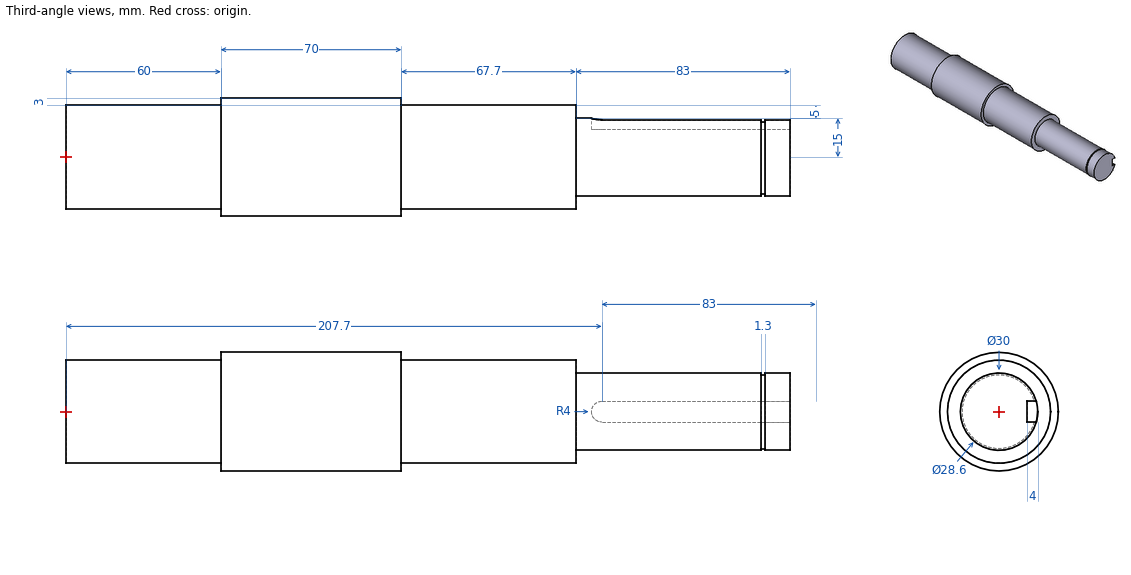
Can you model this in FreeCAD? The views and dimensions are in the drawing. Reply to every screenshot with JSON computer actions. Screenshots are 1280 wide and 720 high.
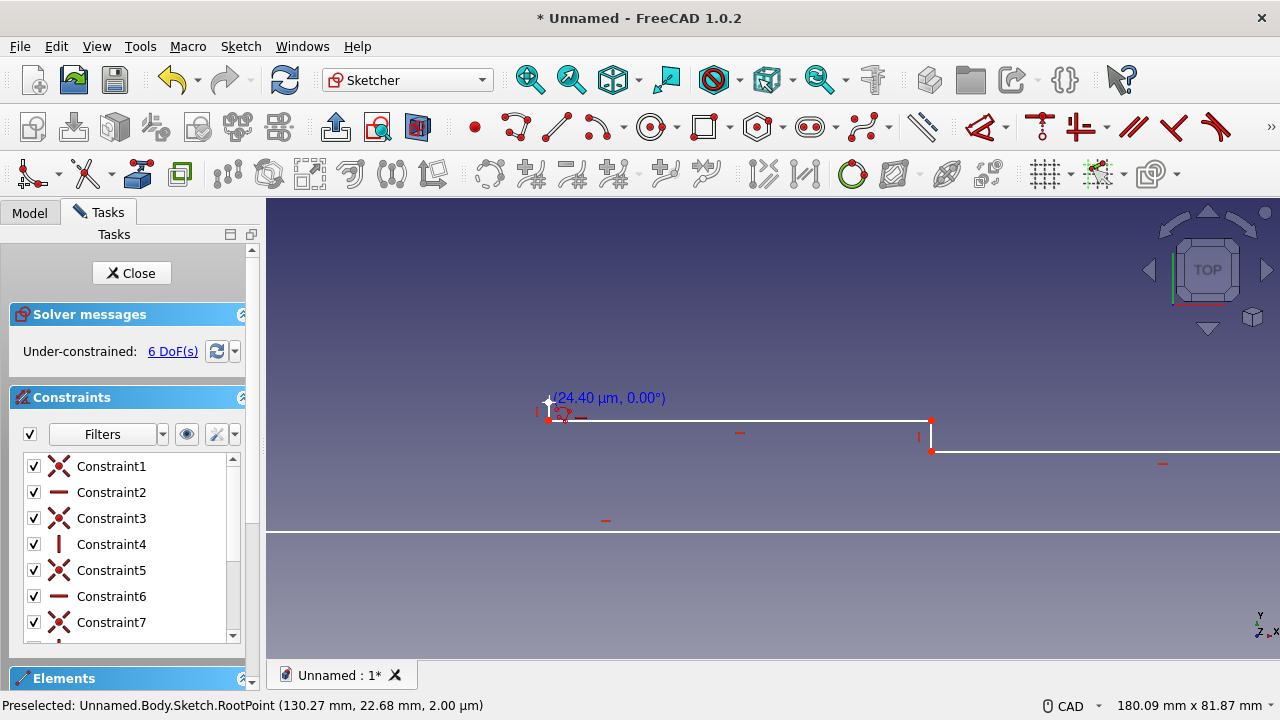
{"action": "scroll", "coordinate": [761, 406], "scroll_direction": "down", "scroll_amount": 5}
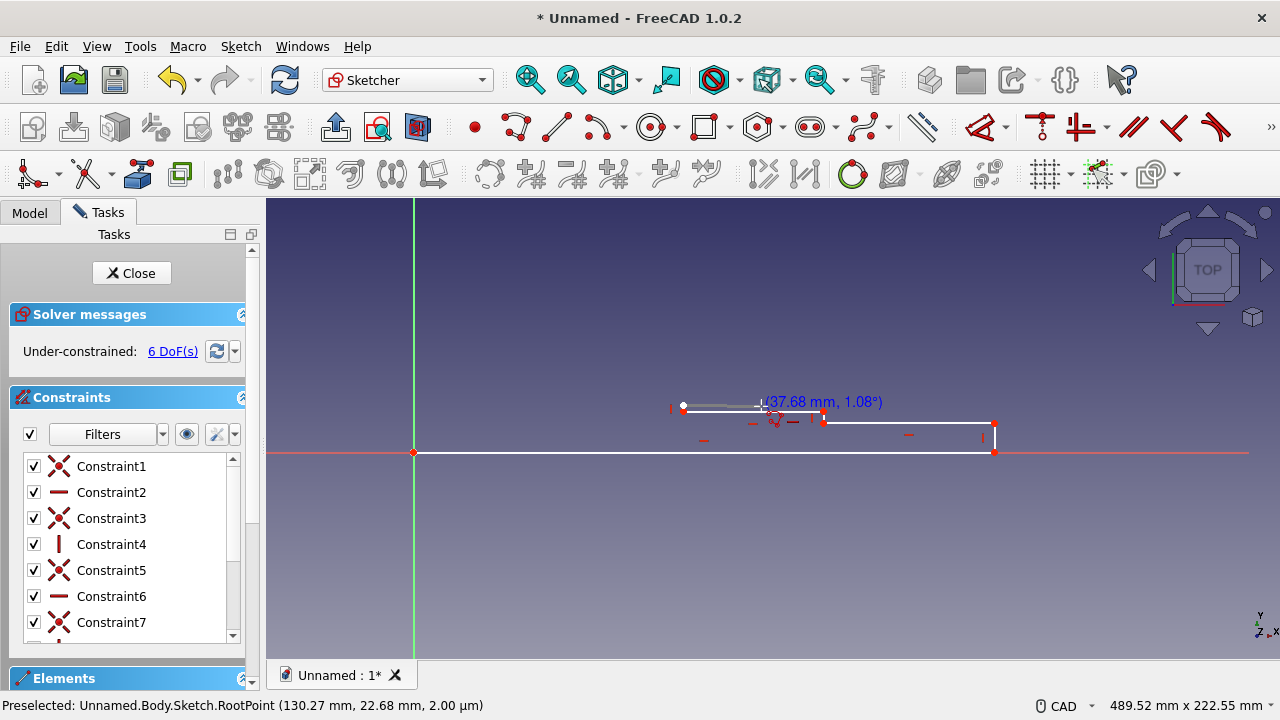
{"action": "left_click", "coordinate": [538, 405]}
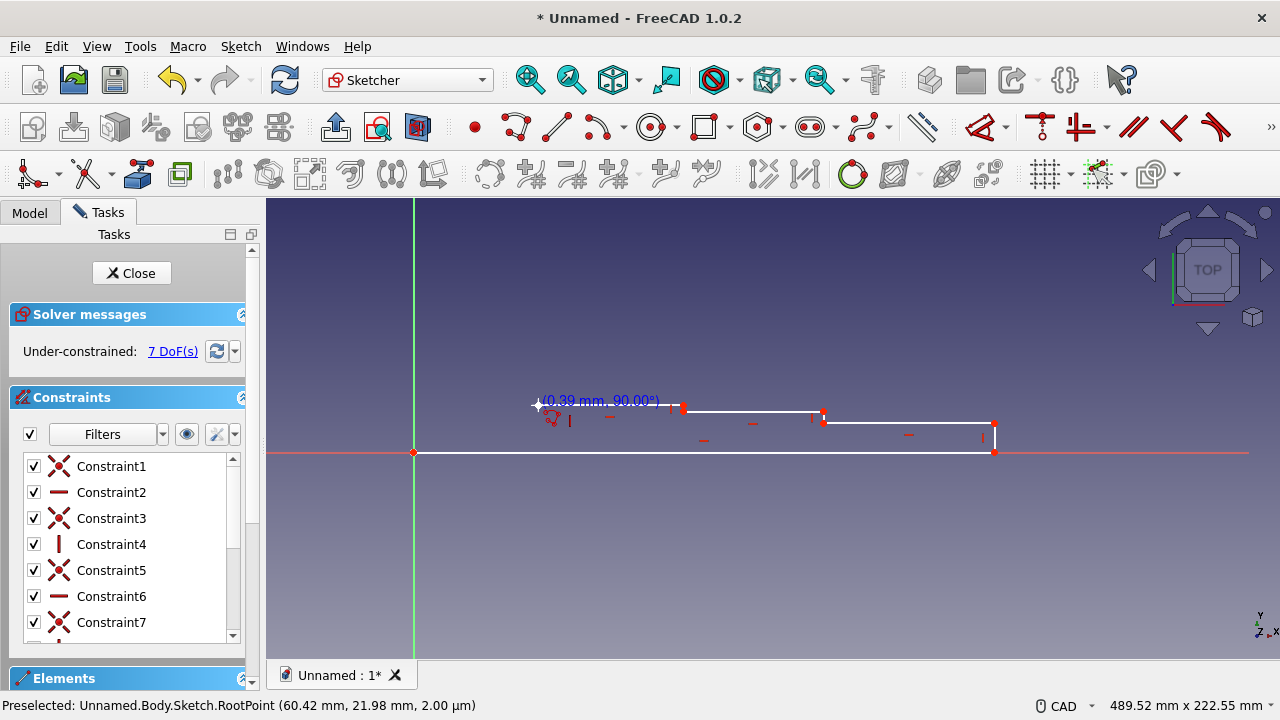
{"action": "scroll", "coordinate": [538, 411], "scroll_direction": "up", "scroll_amount": 5}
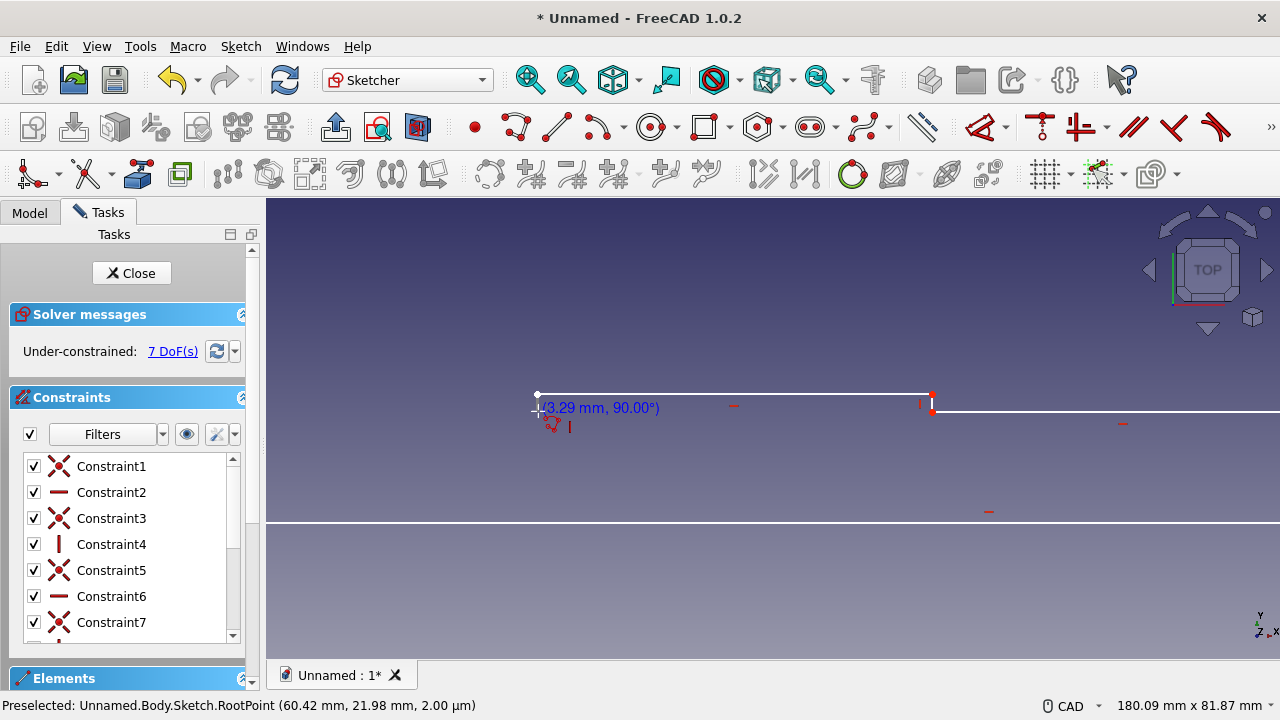
{"action": "left_click", "coordinate": [538, 410]}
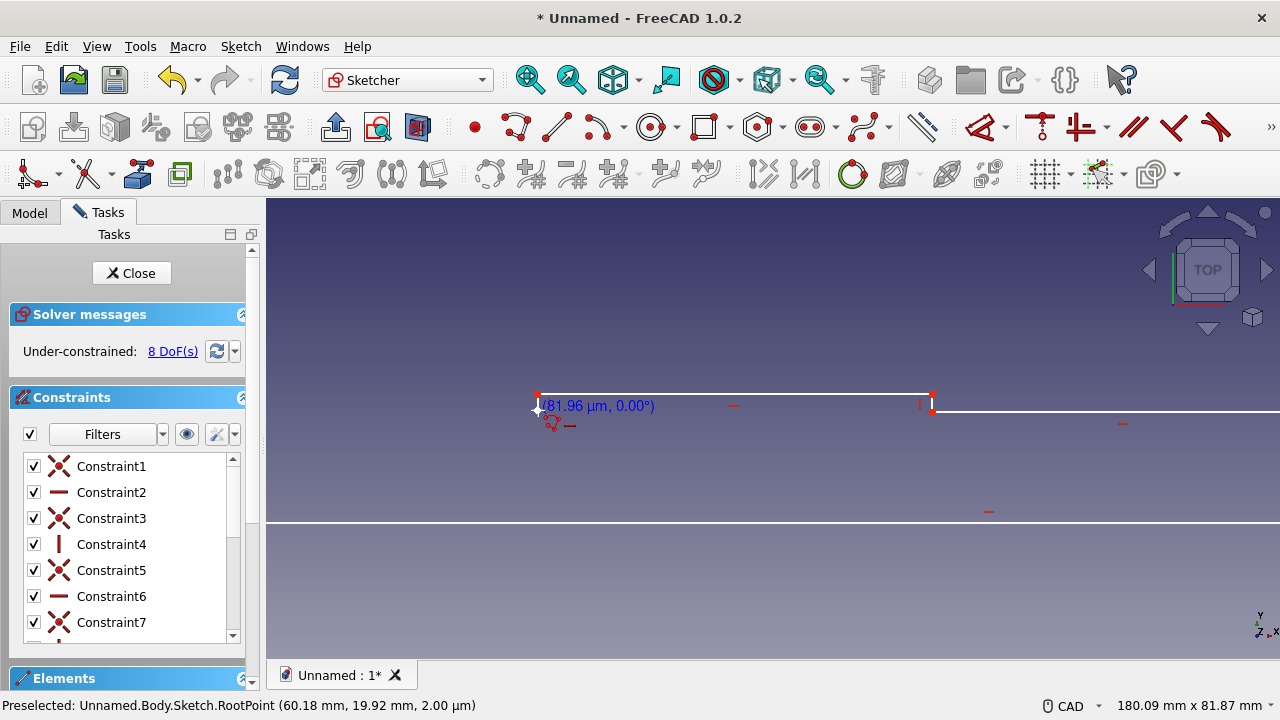
{"action": "scroll", "coordinate": [538, 411], "scroll_direction": "down", "scroll_amount": 5}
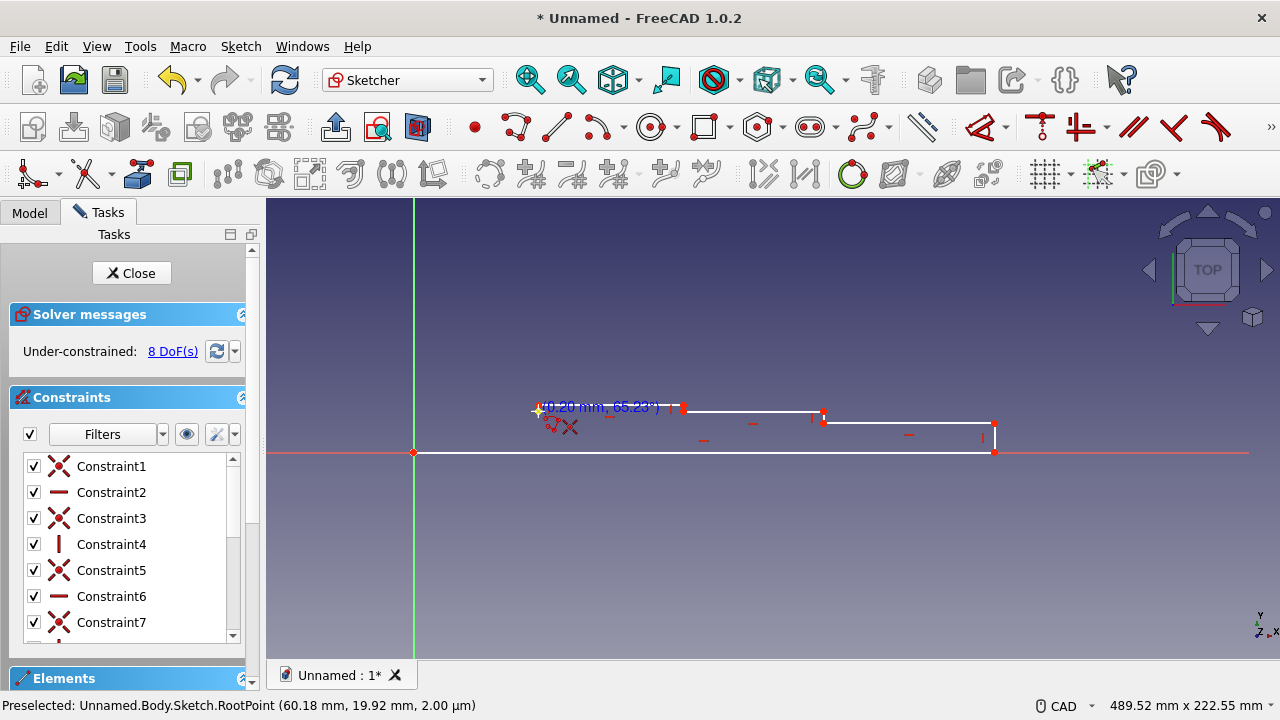
{"action": "left_click", "coordinate": [423, 411]}
{"action": "left_click", "coordinate": [414, 453]}
{"action": "key", "text": "Escape"}
{"action": "key", "text": "Escape"}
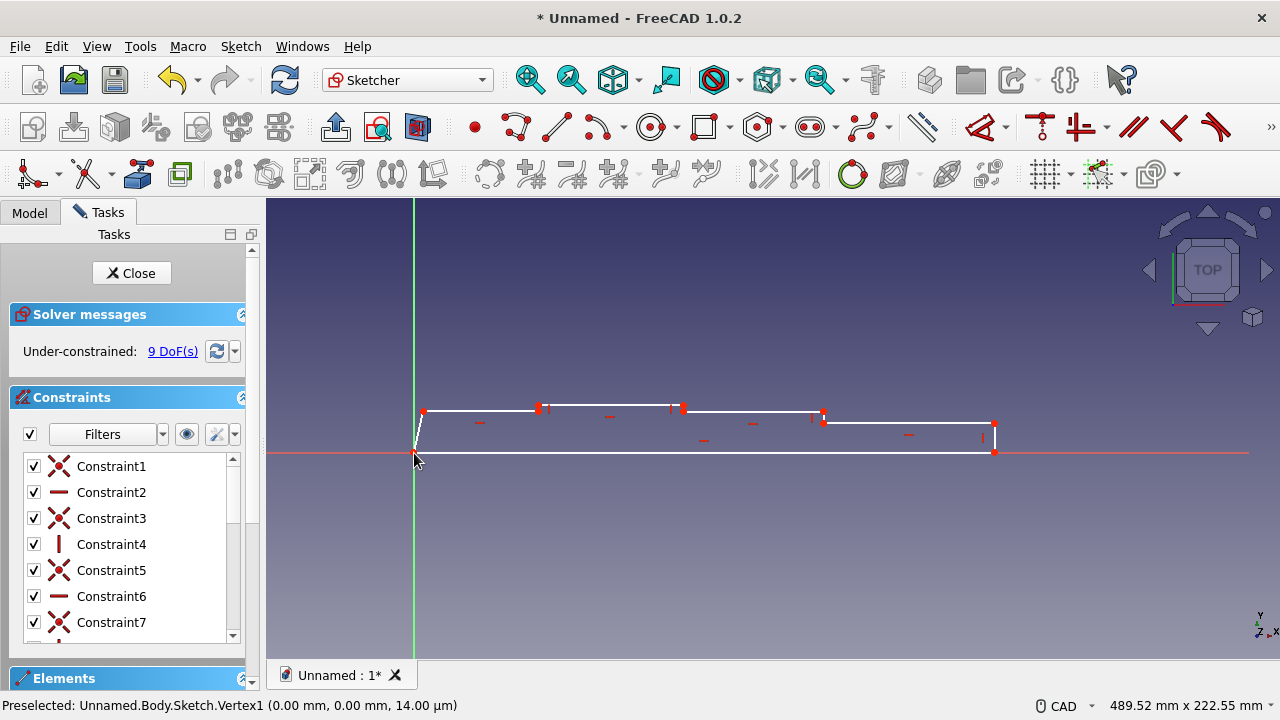
{"action": "left_click", "coordinate": [417, 440]}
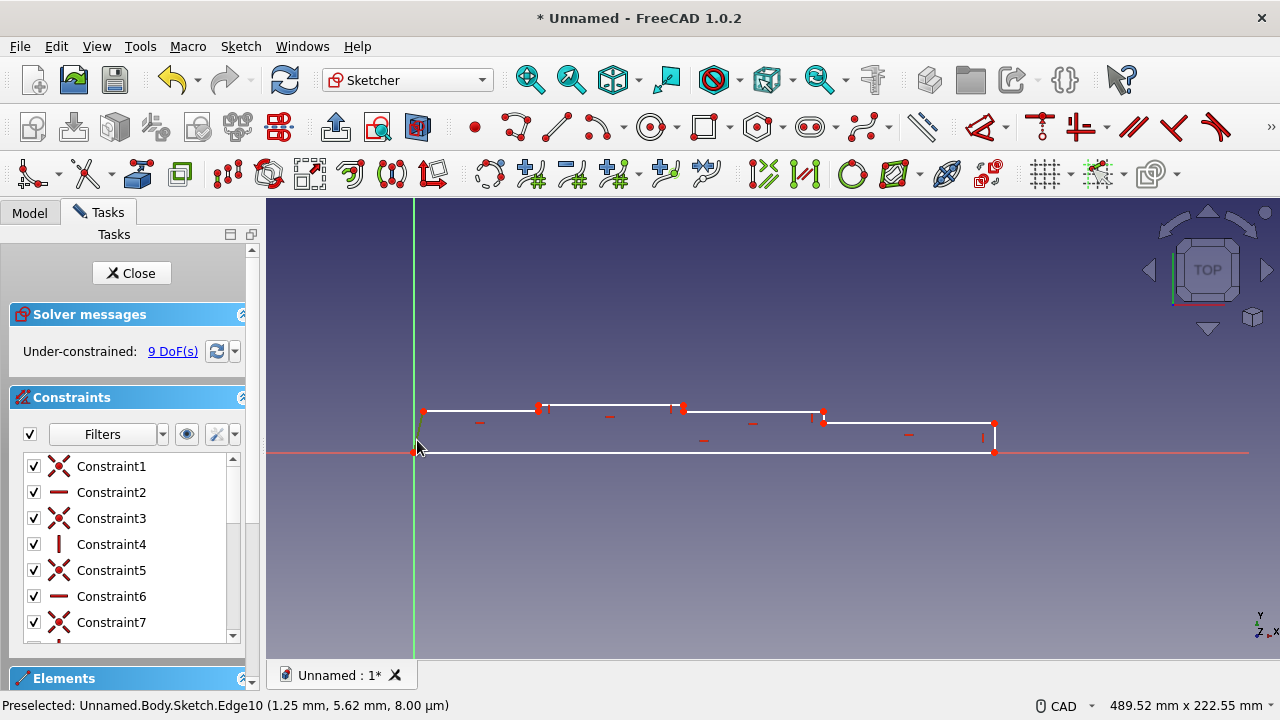
{"action": "key", "text": "v"}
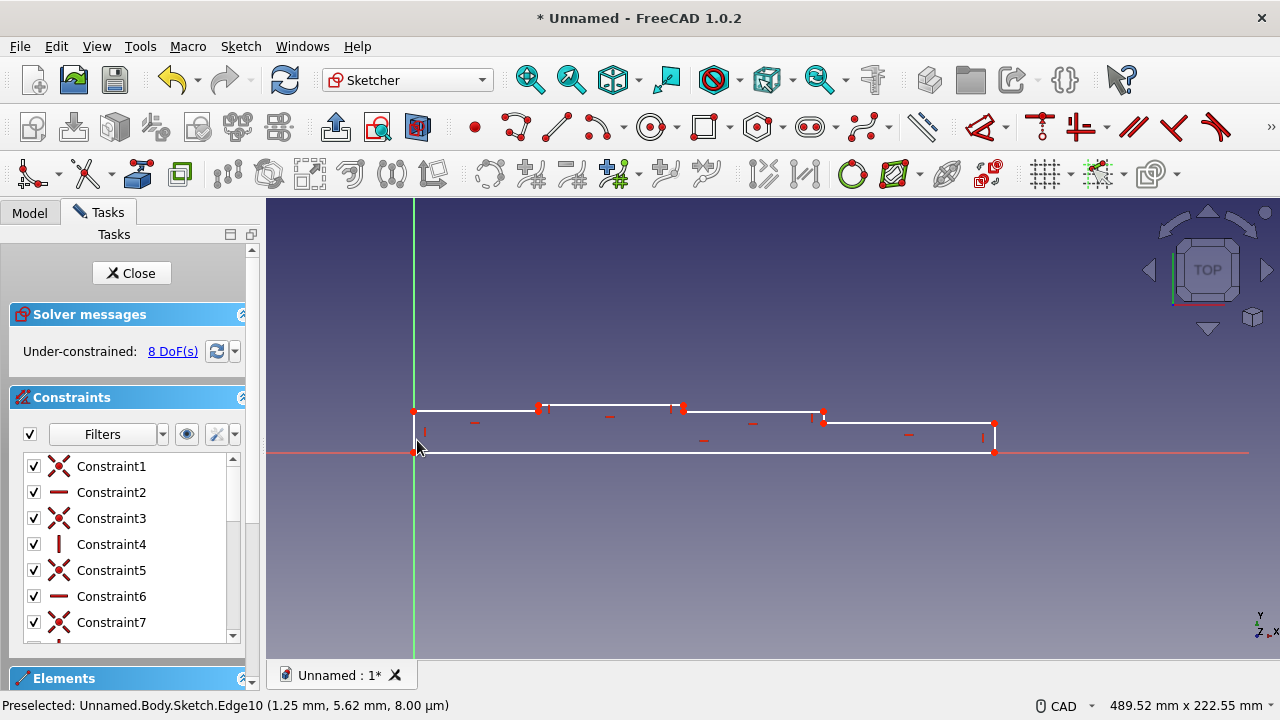
{"action": "left_click", "coordinate": [980, 128]}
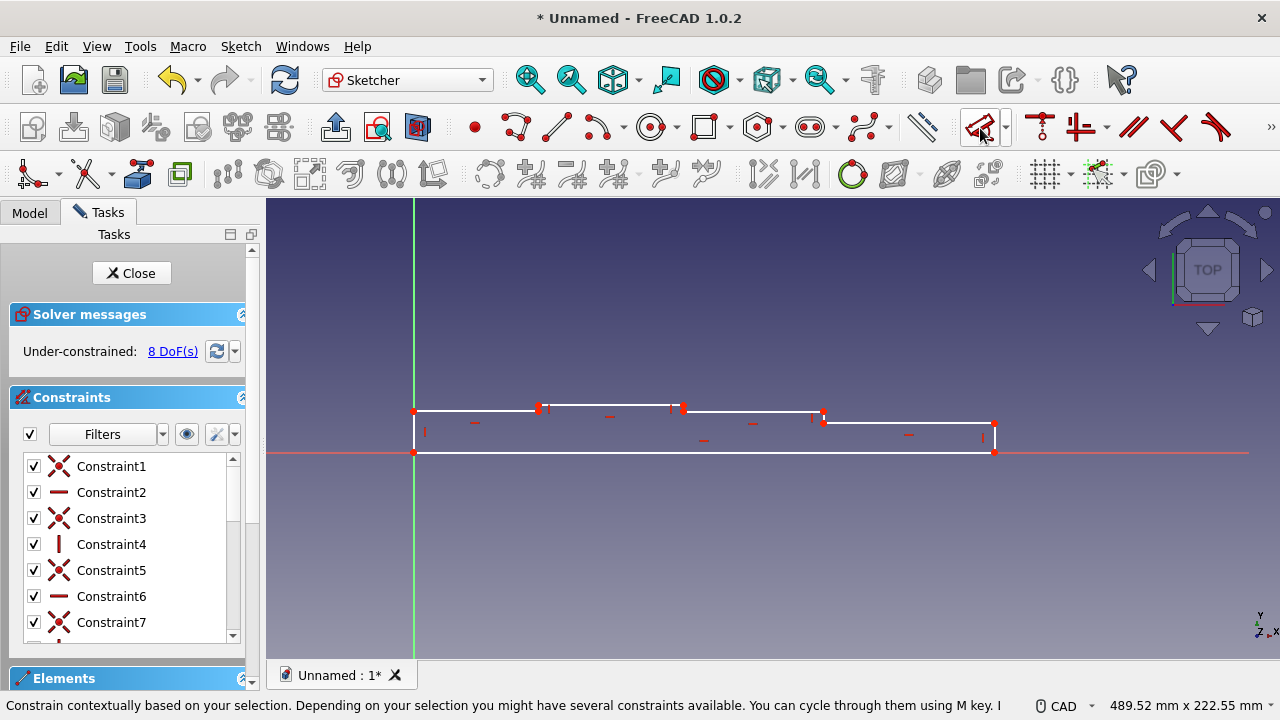
{"action": "scroll", "coordinate": [824, 417], "scroll_direction": "up", "scroll_amount": 7}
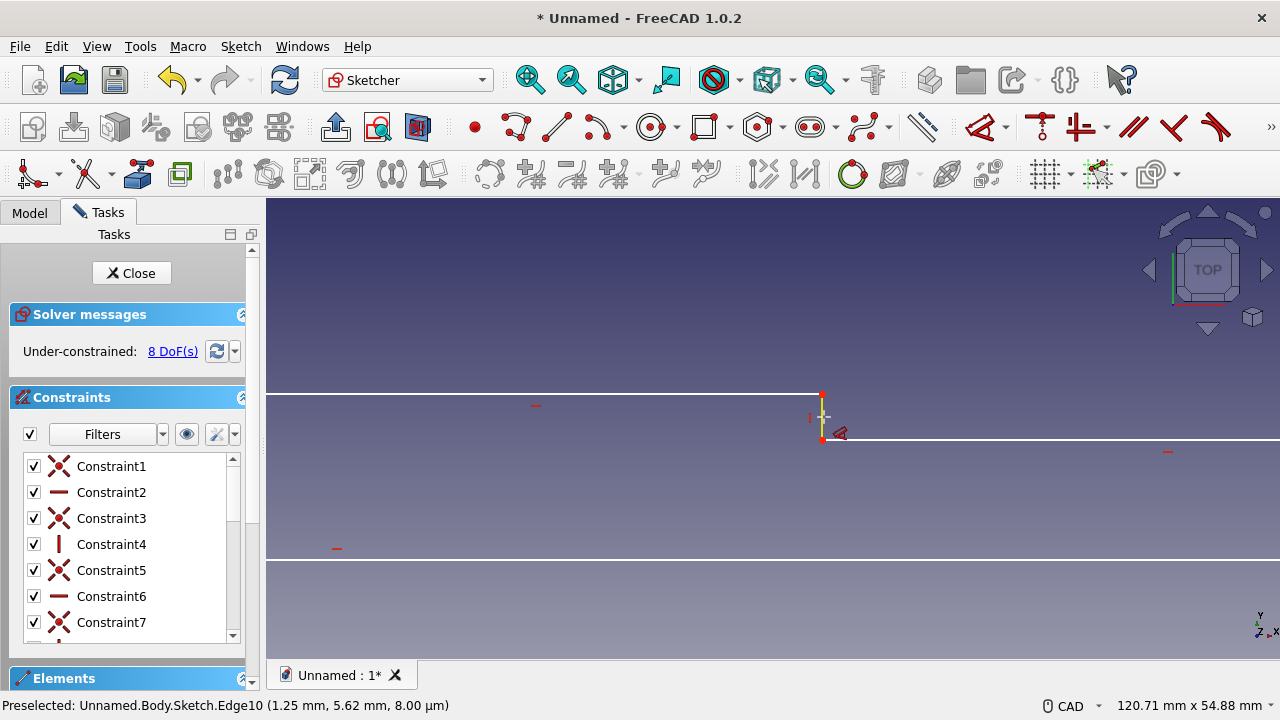
{"action": "left_click", "coordinate": [822, 417]}
{"action": "left_click", "coordinate": [856, 417]}